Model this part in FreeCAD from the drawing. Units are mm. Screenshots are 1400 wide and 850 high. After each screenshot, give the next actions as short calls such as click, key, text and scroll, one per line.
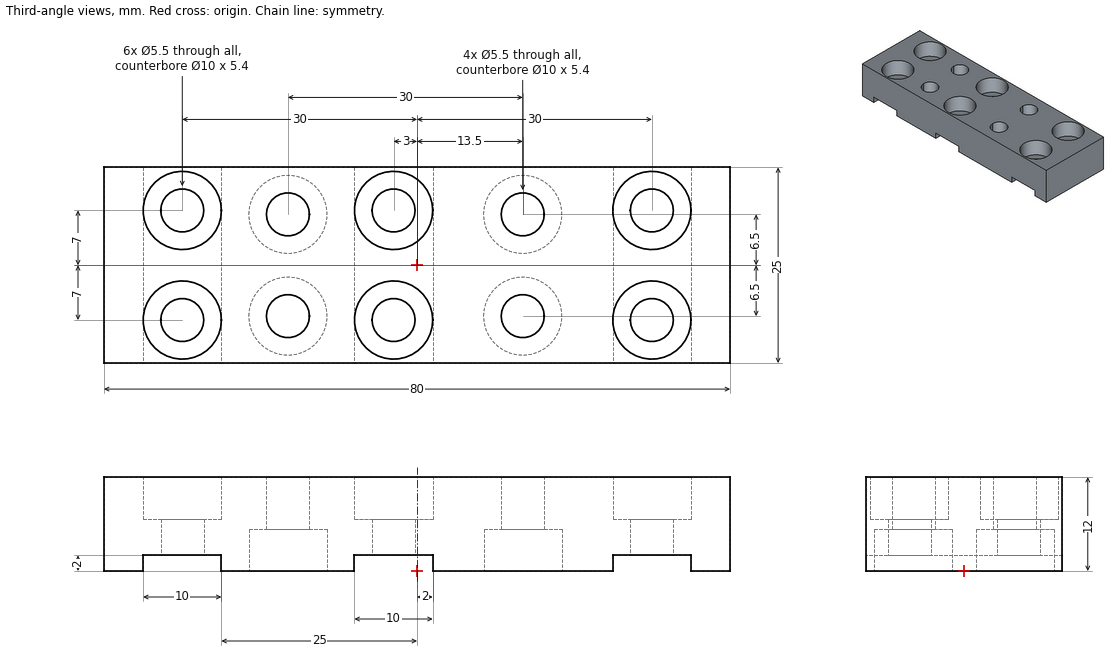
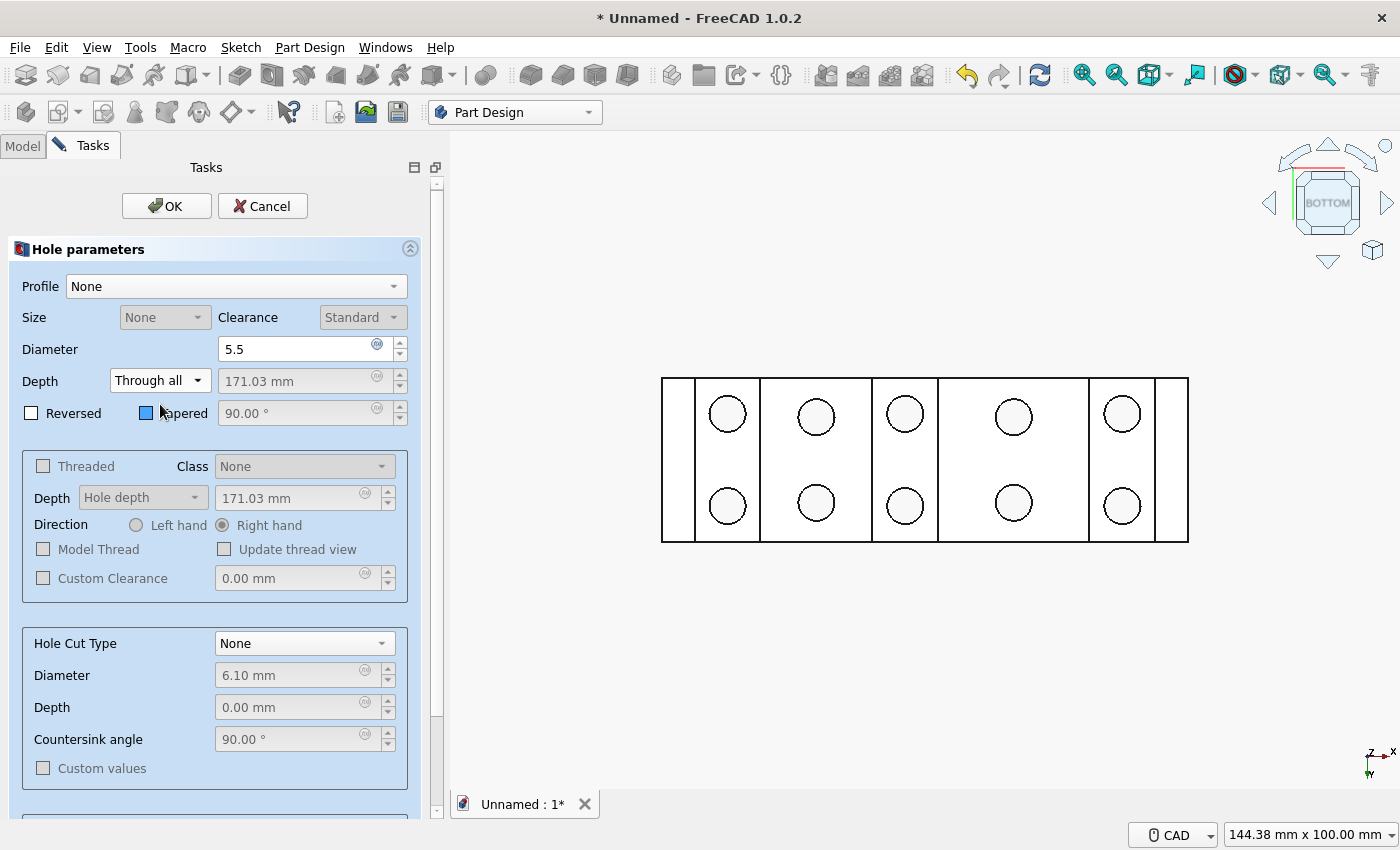
click(306, 644)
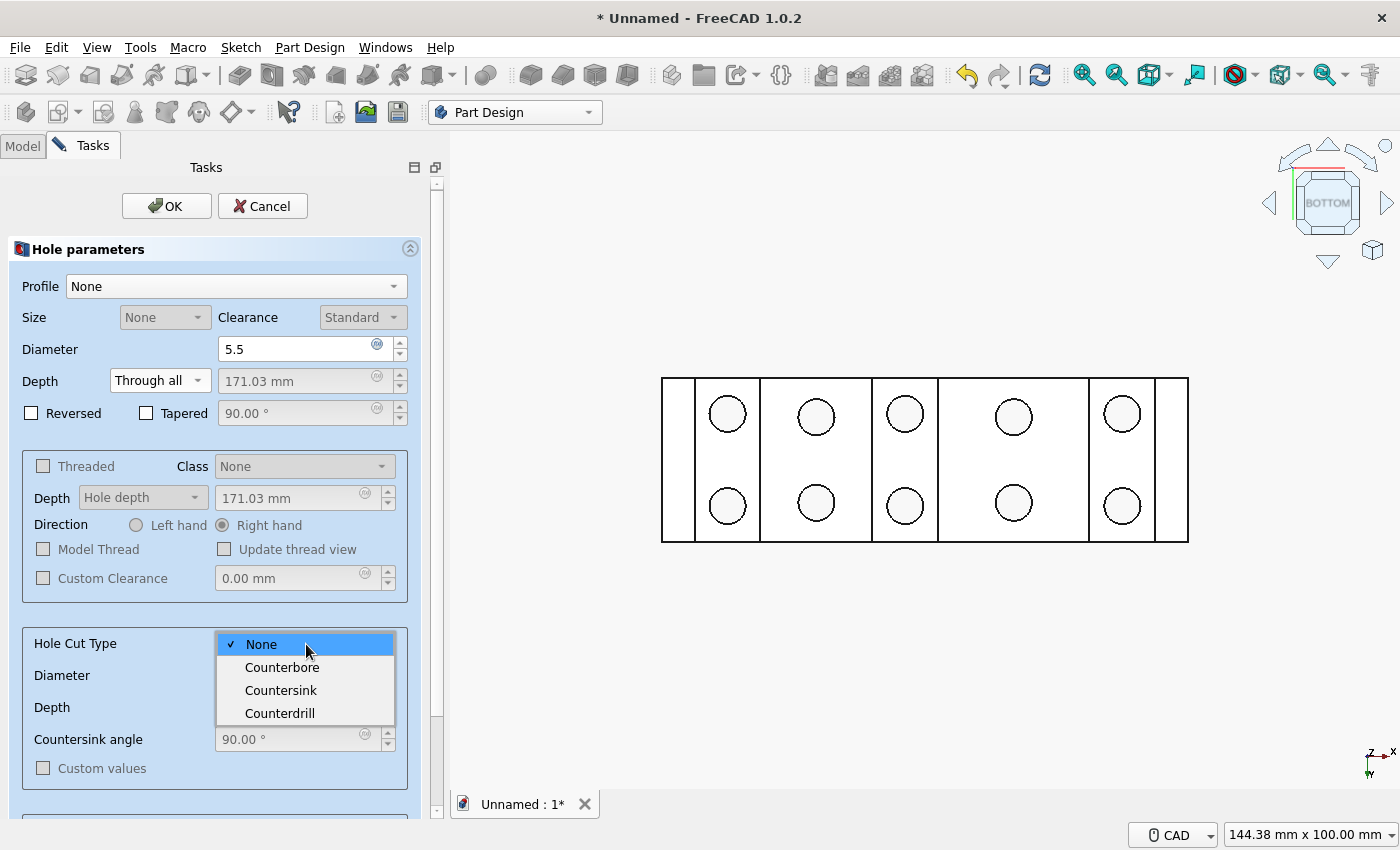
click(304, 668)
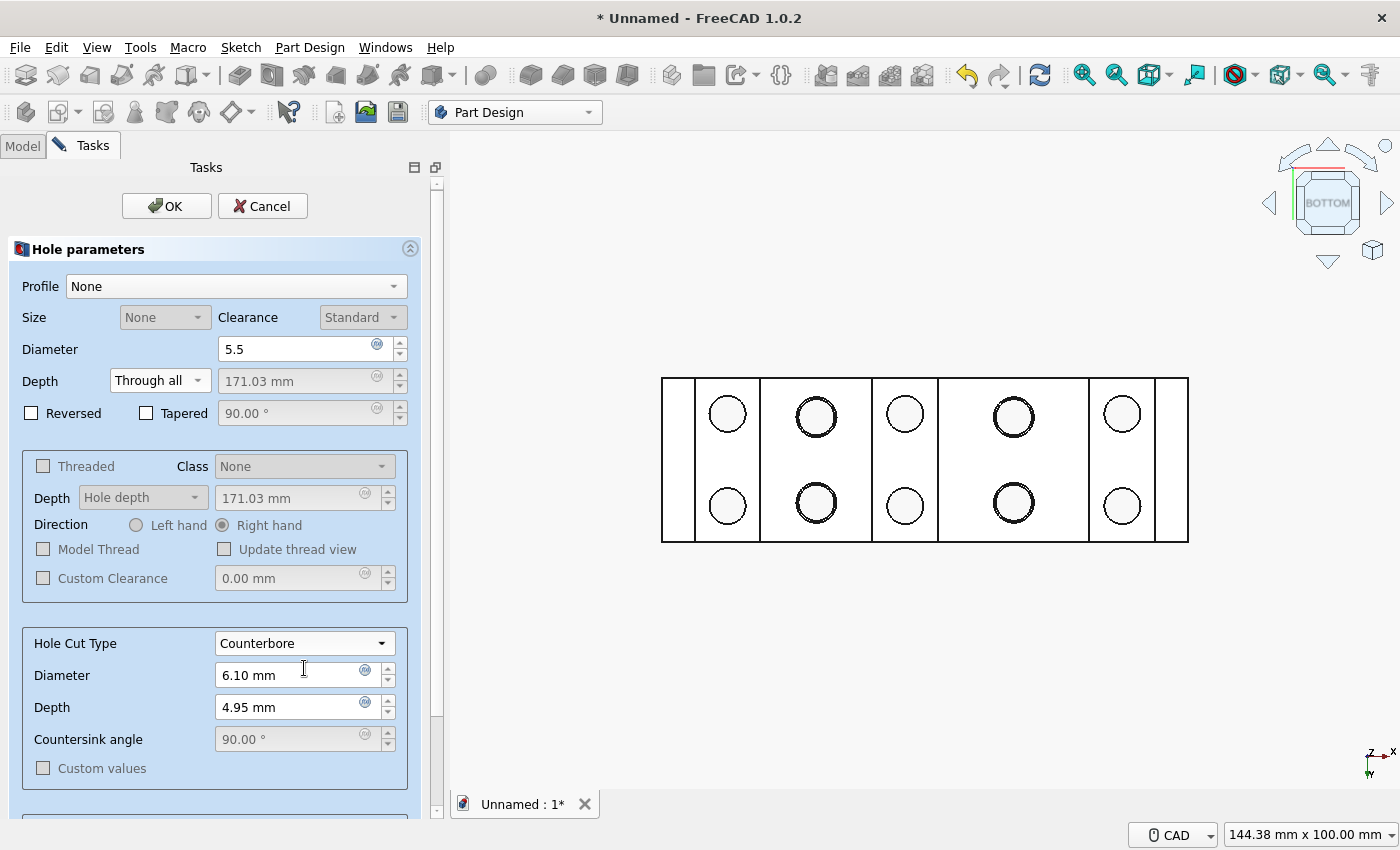
triple_click(298, 675)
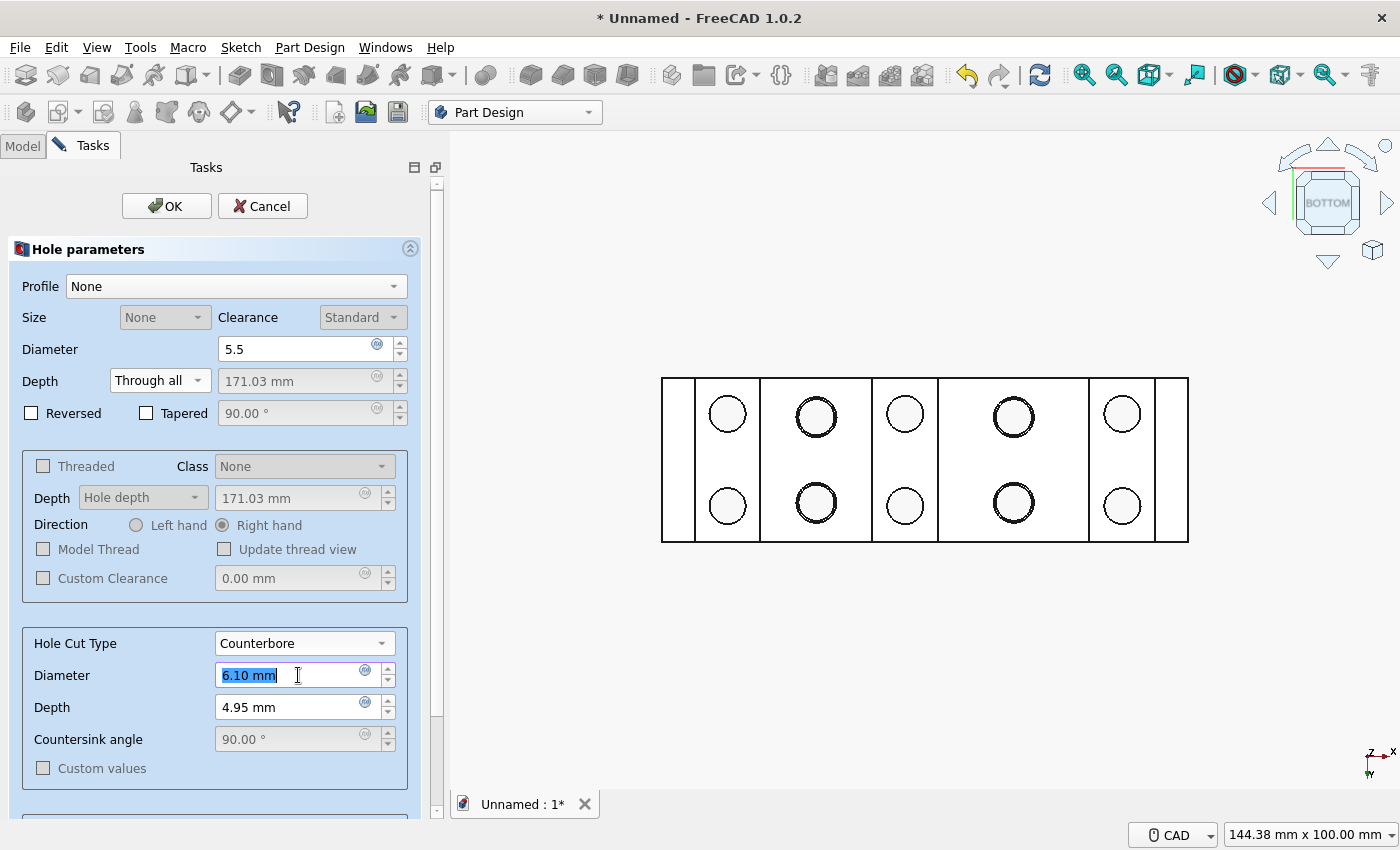
text(10)
key(Tab)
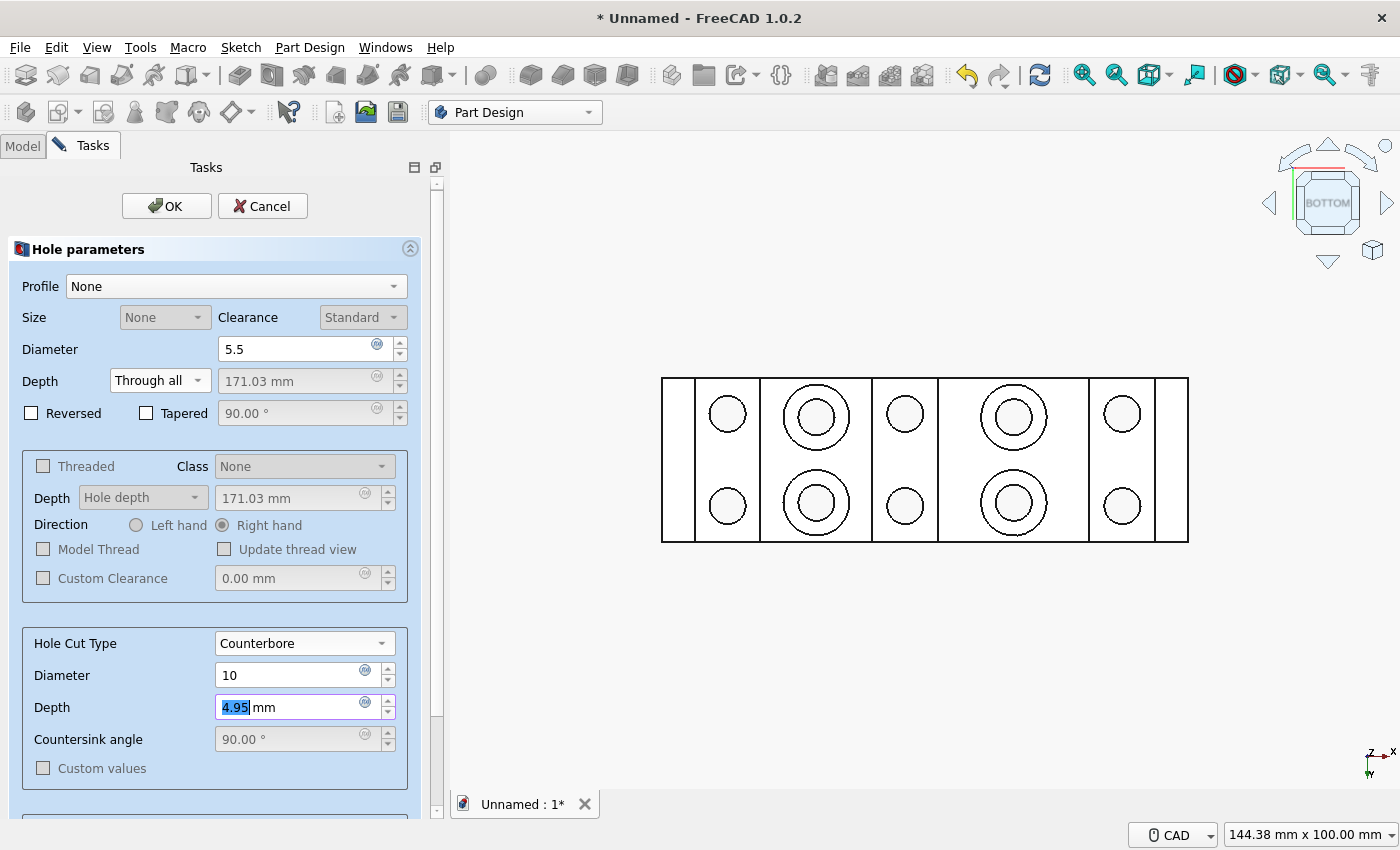
text(5.4)
key(Tab)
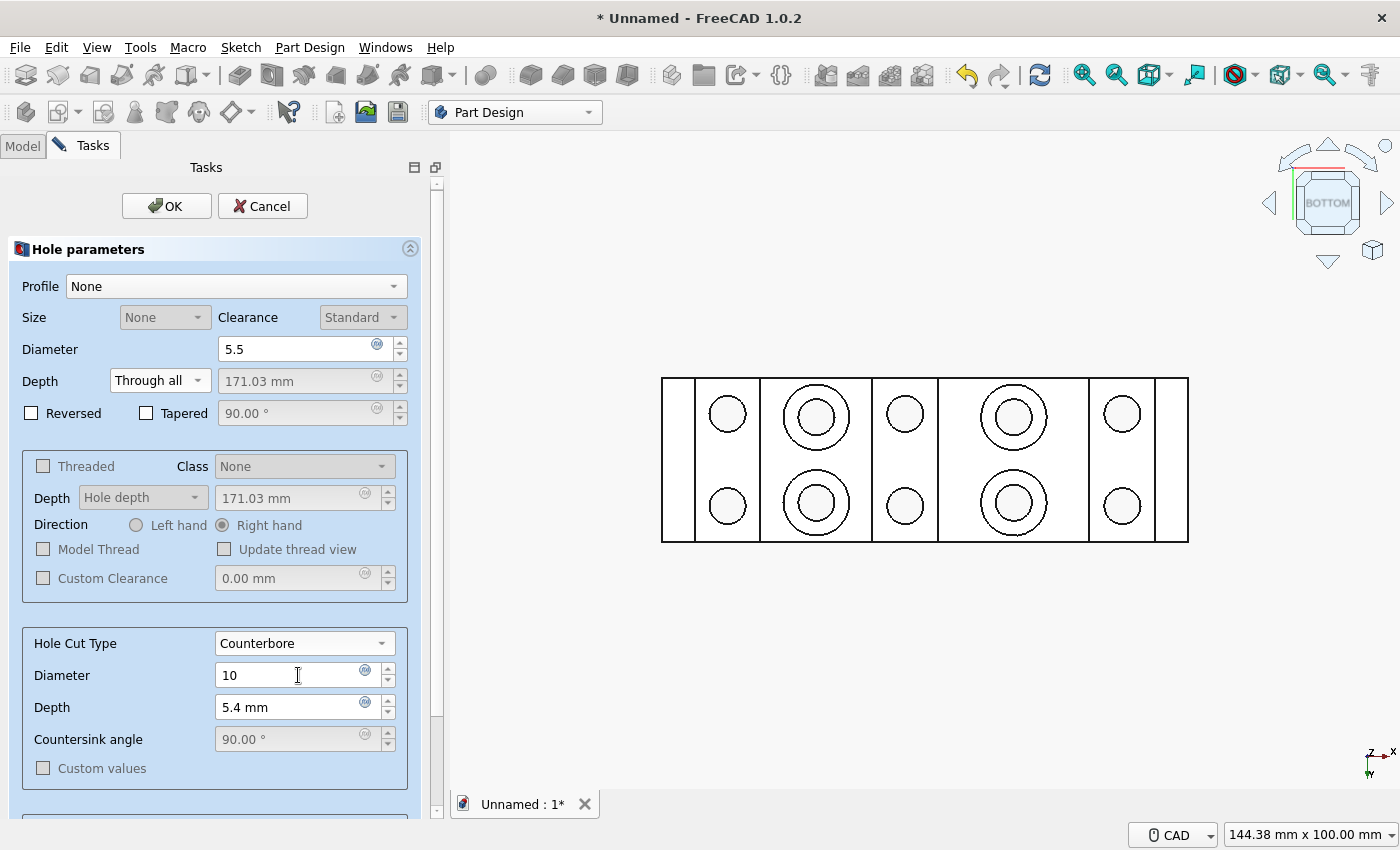
click(167, 206)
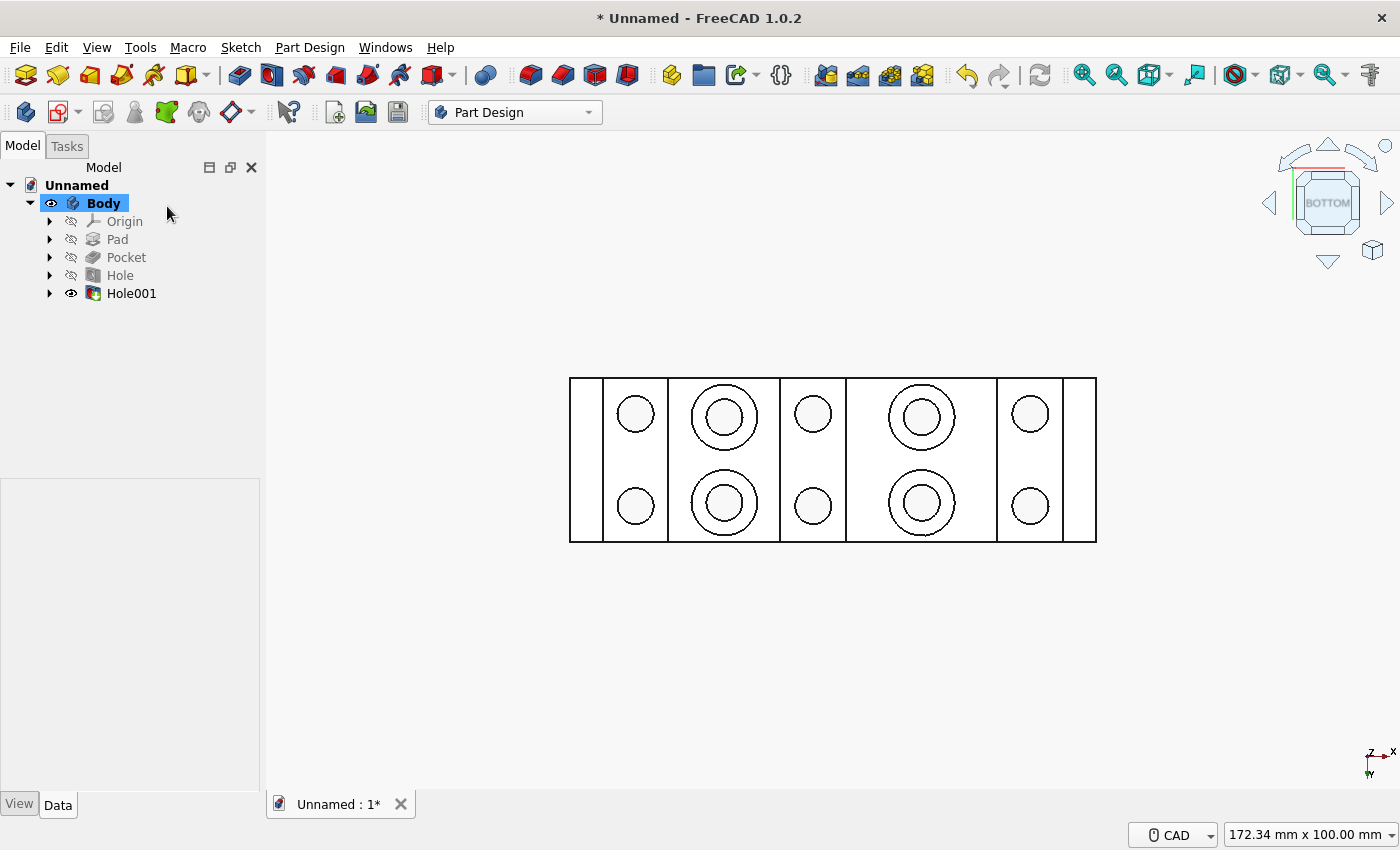
key(0)